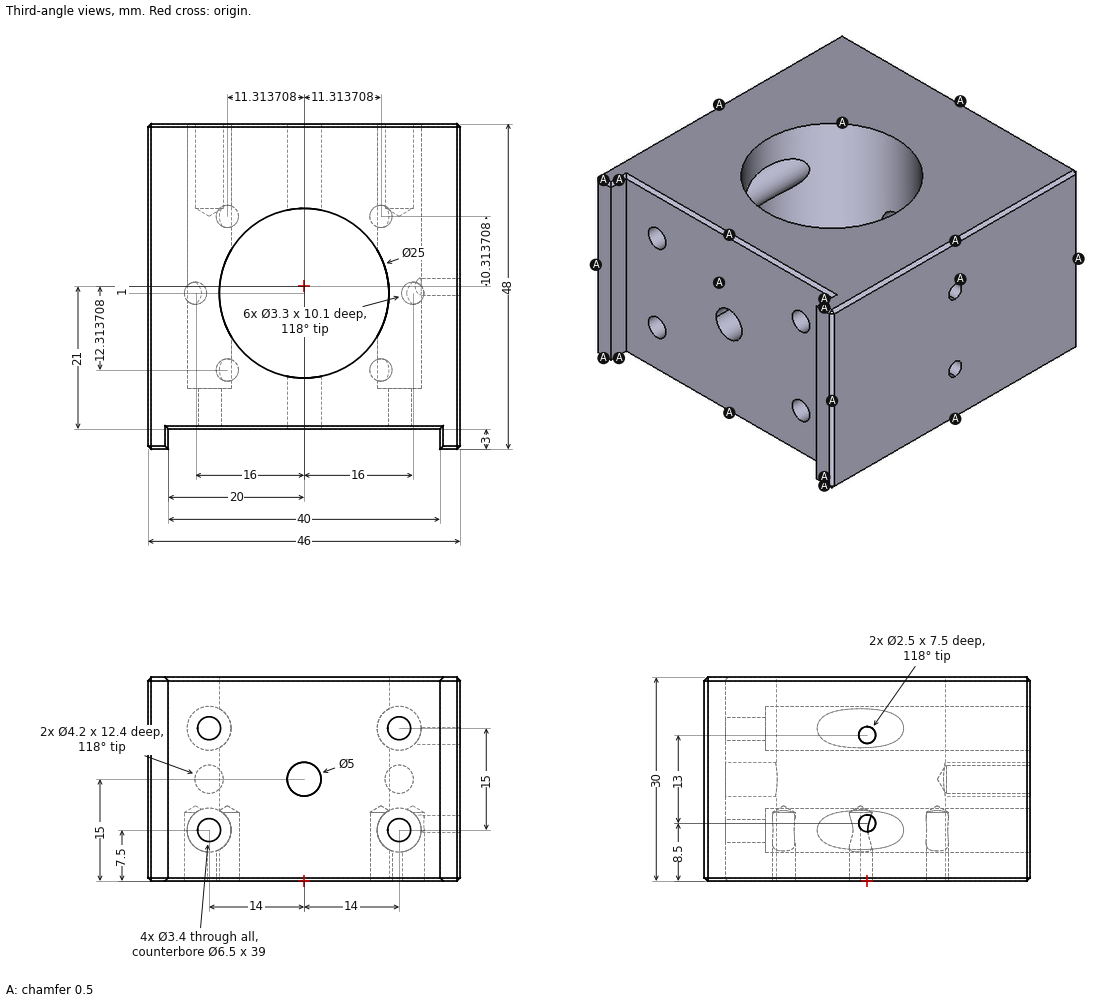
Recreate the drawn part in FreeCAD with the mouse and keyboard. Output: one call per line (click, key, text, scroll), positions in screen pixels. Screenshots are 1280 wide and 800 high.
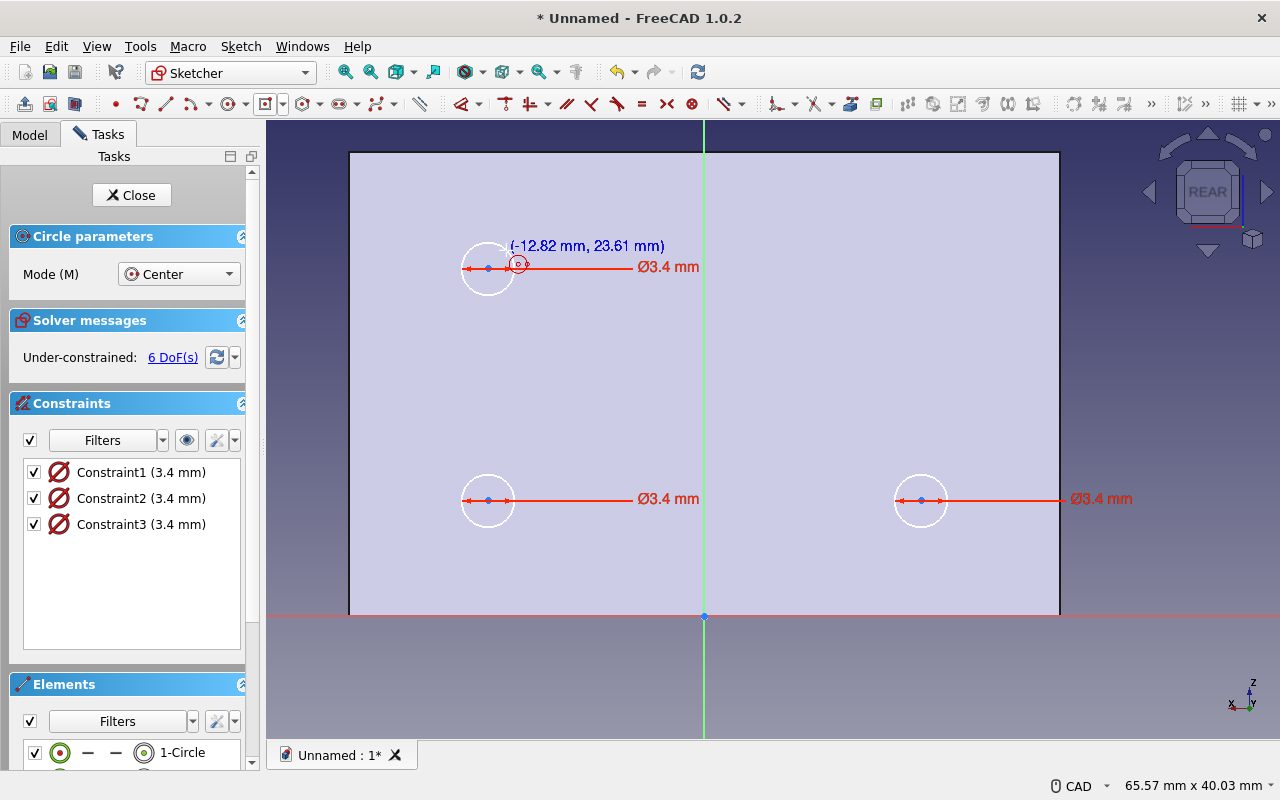
click(921, 268)
move(939, 250)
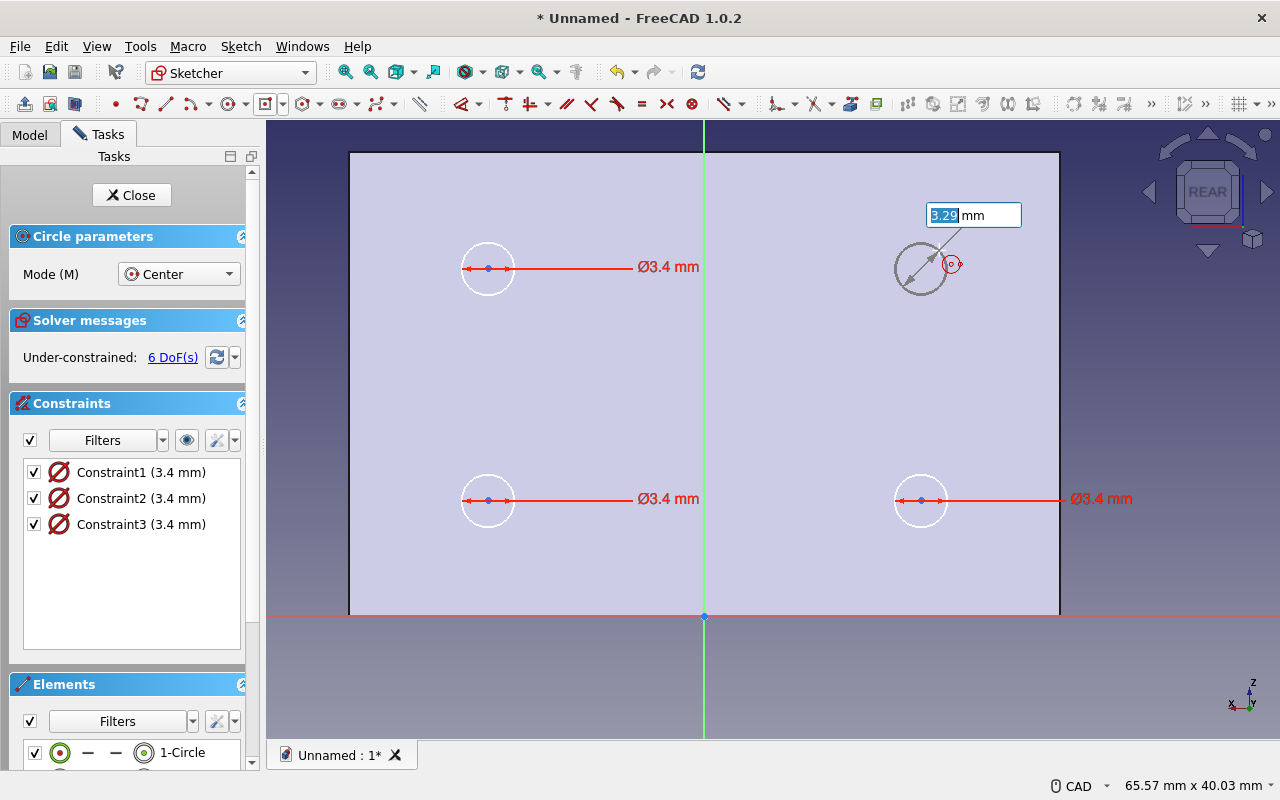
text(3.4)
key(Return)
key(Escape)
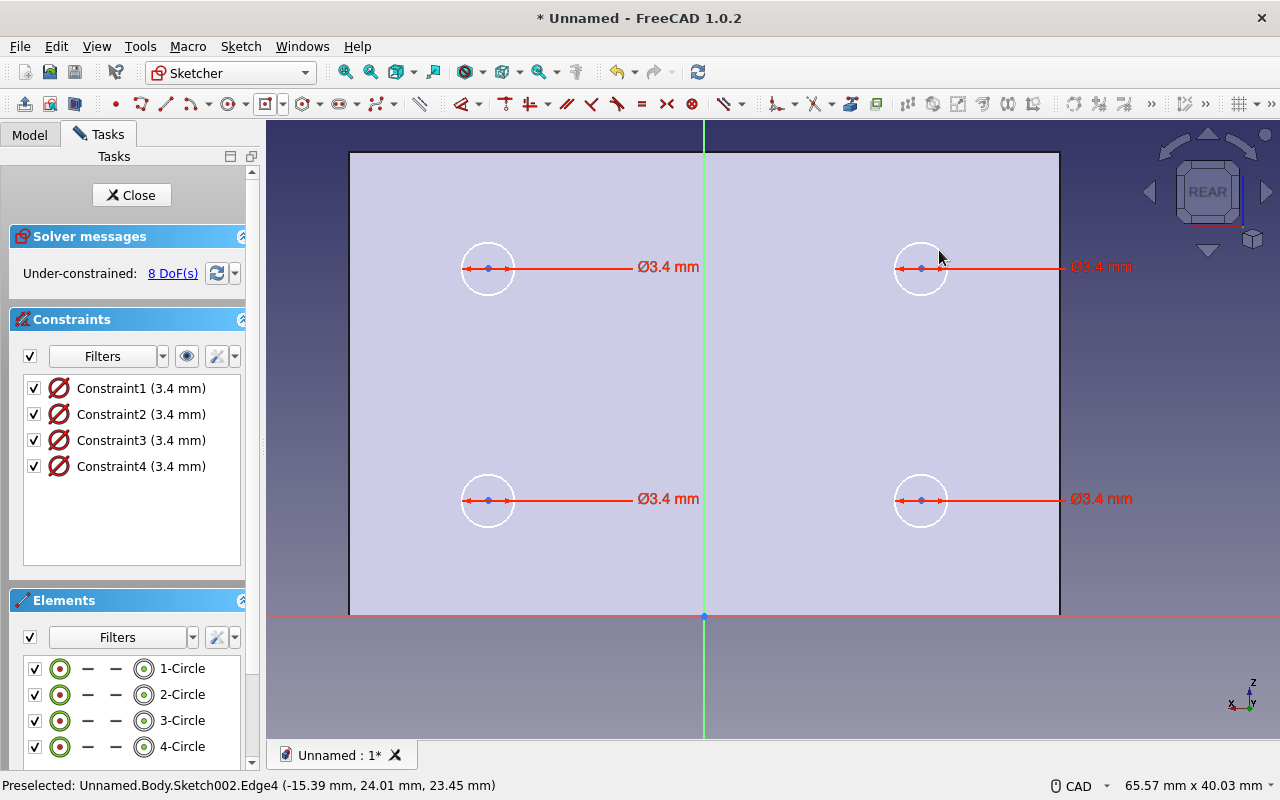
click(921, 501)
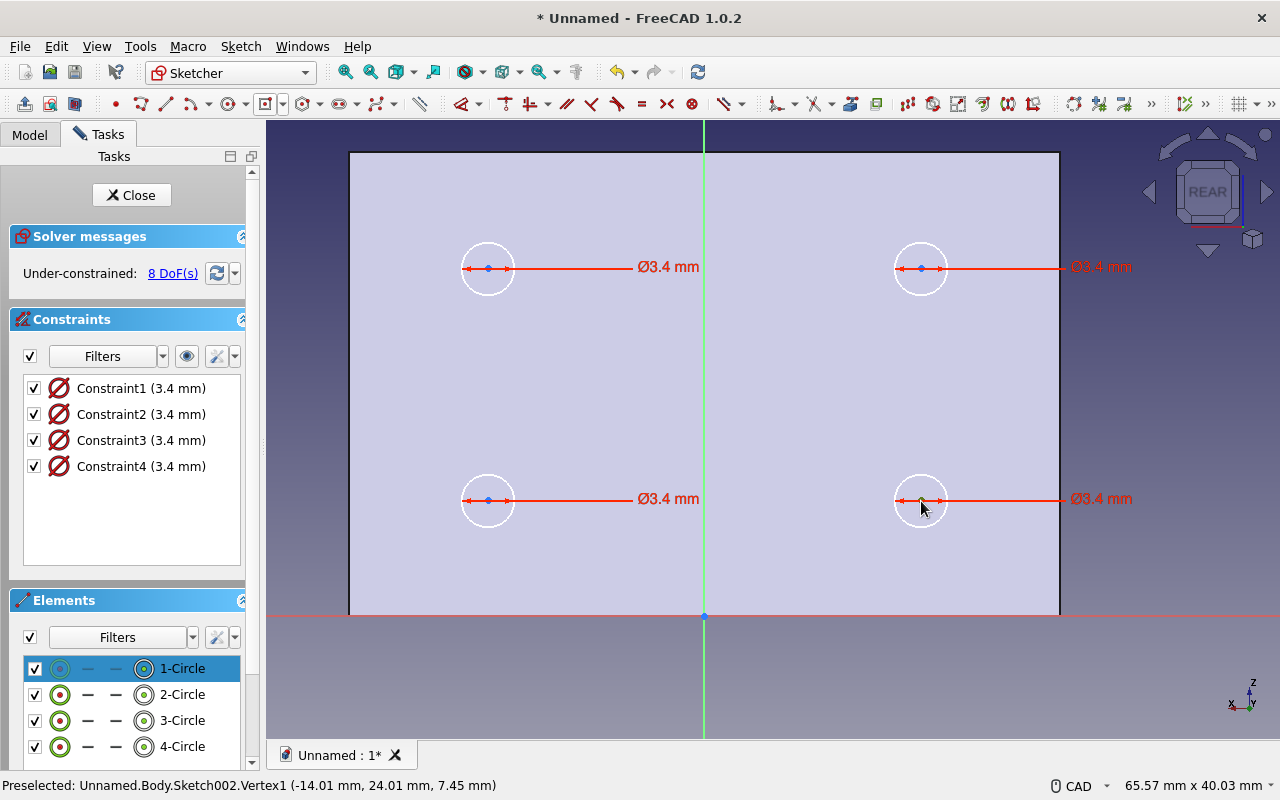
click(488, 501)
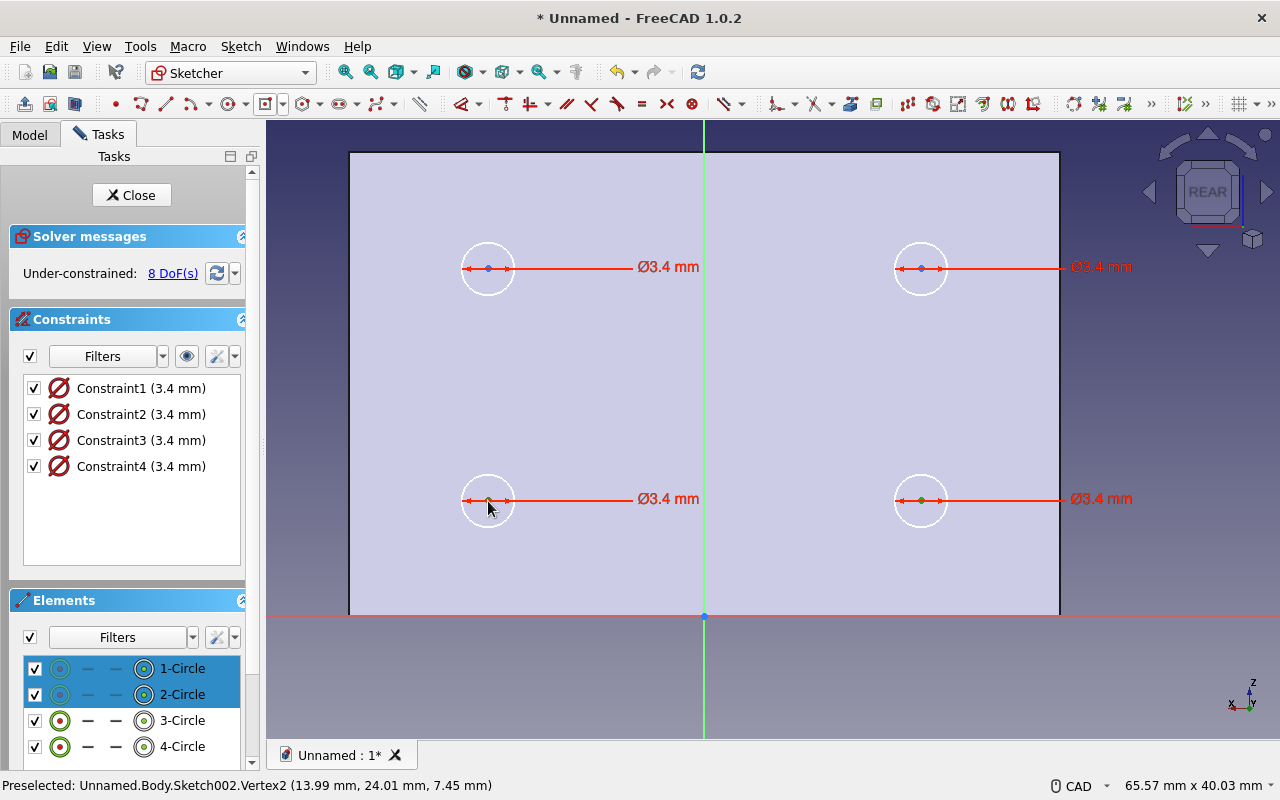
key(h)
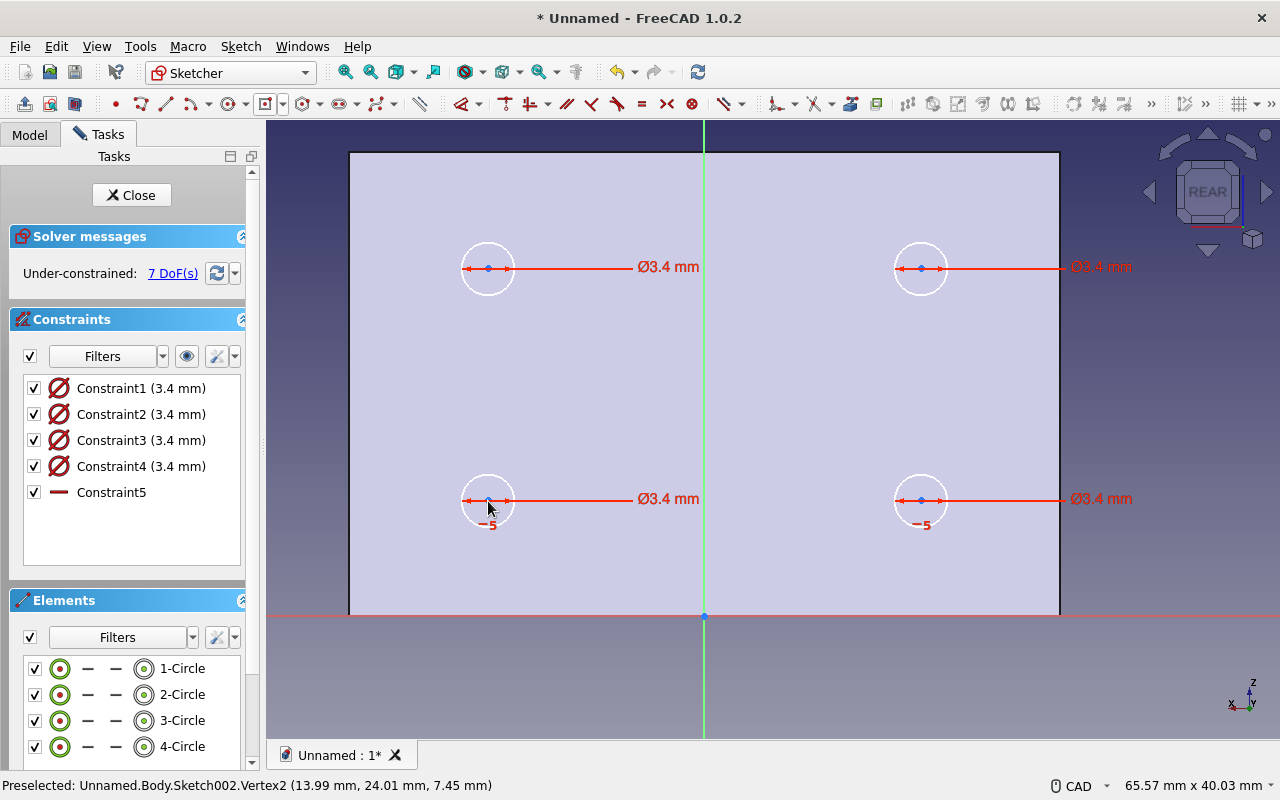
click(488, 501)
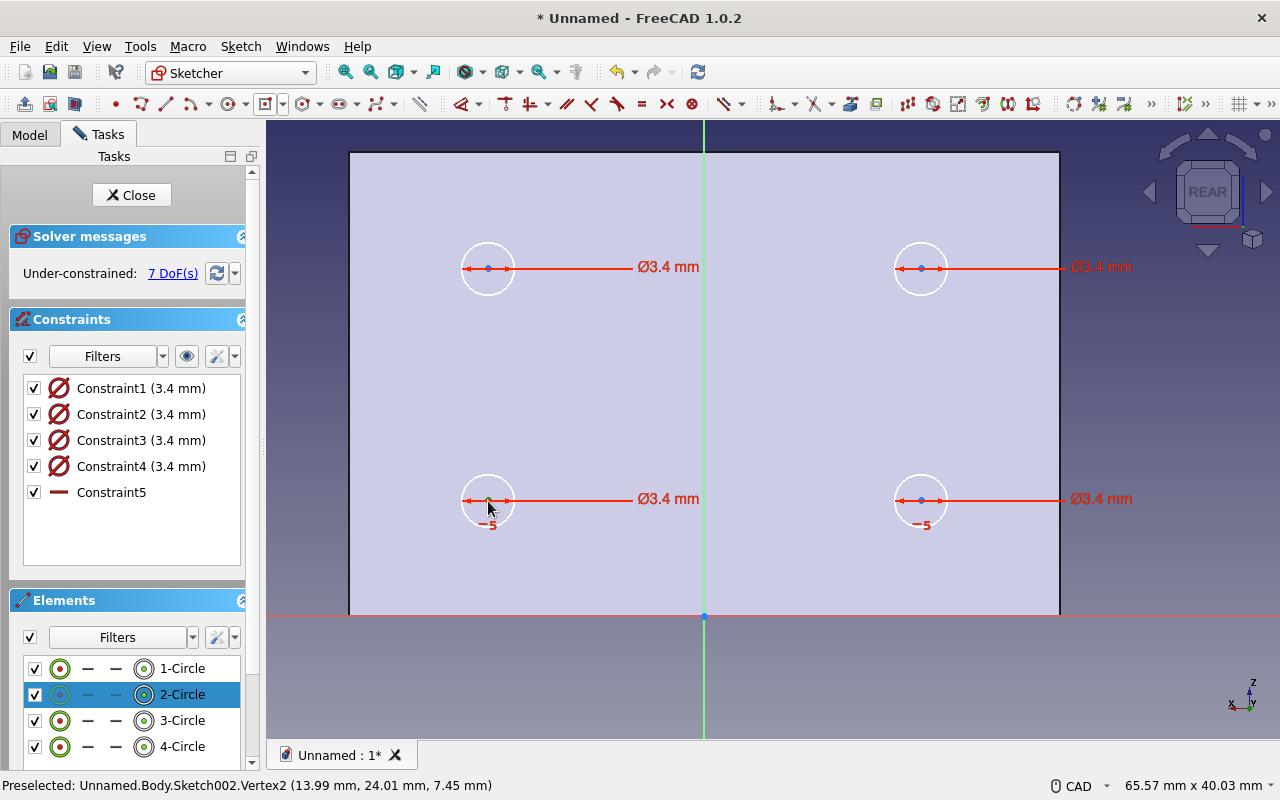
click(488, 269)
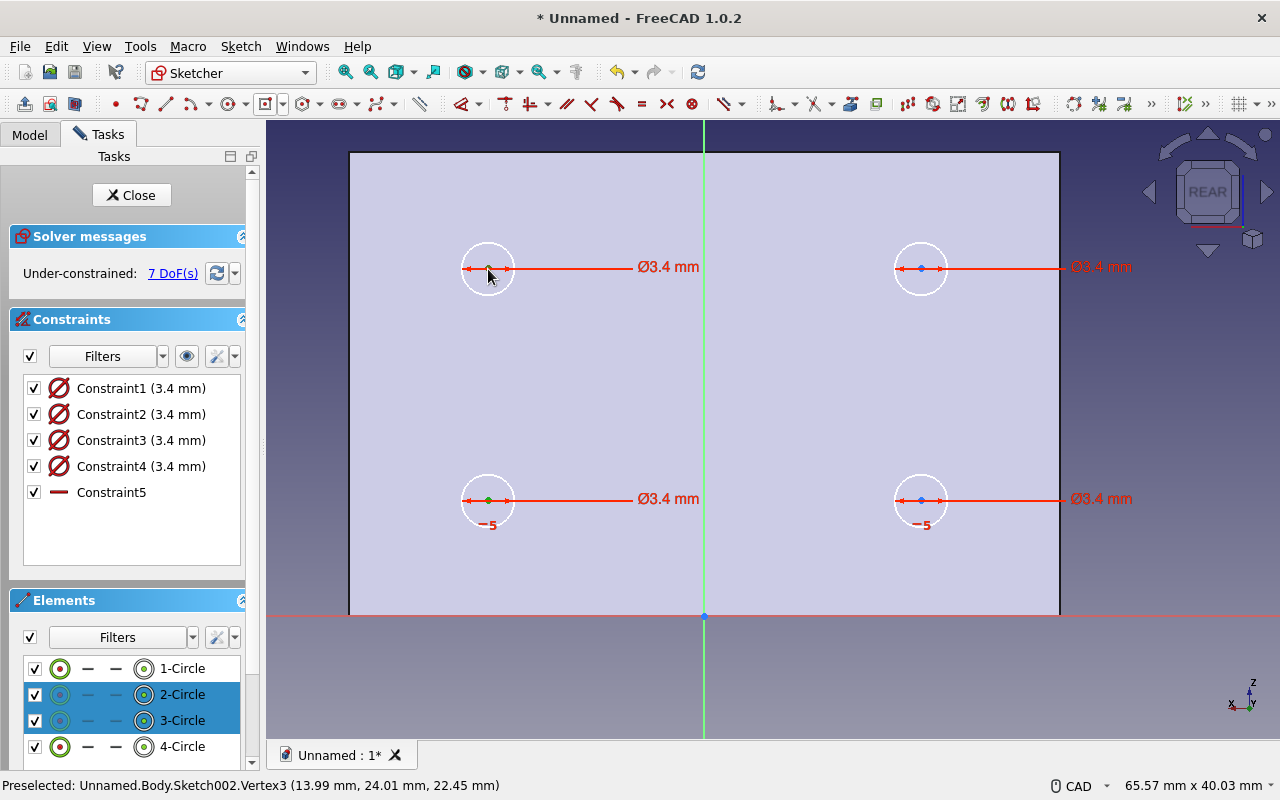
click(548, 104)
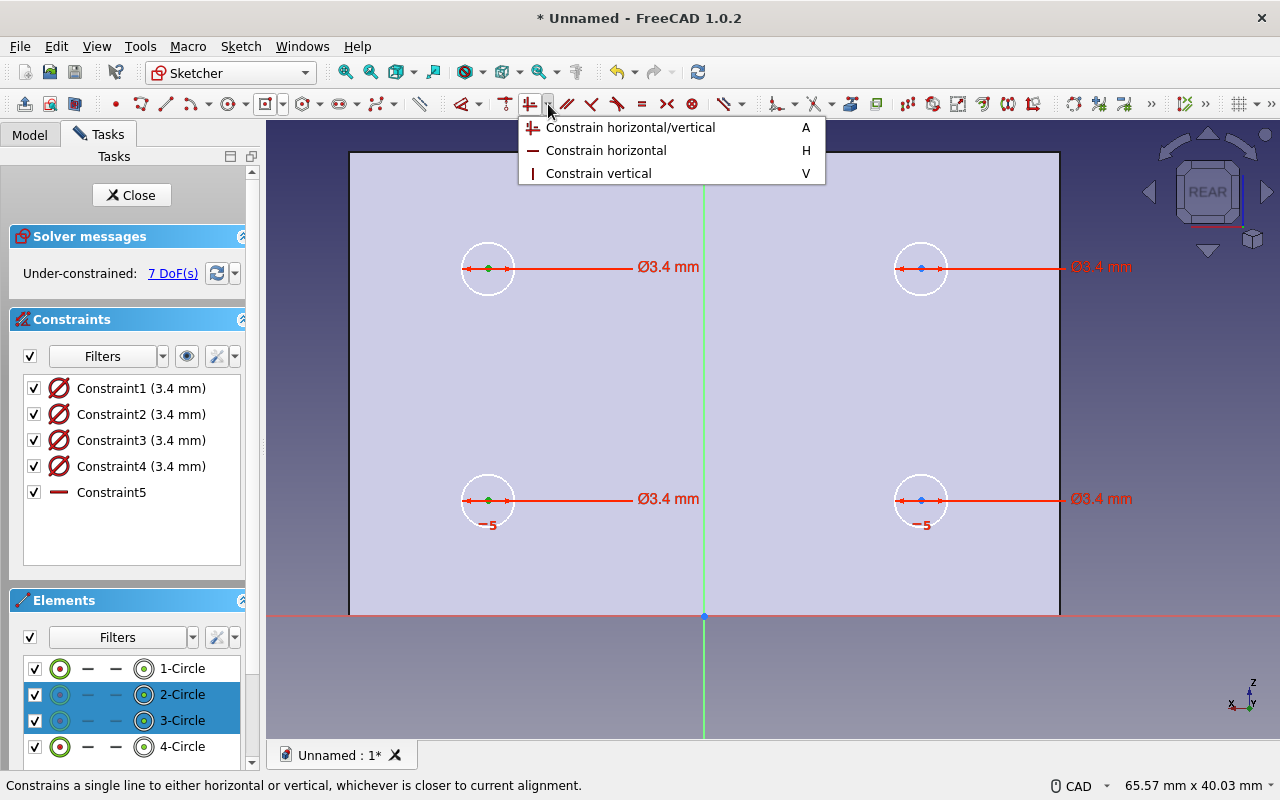
click(672, 174)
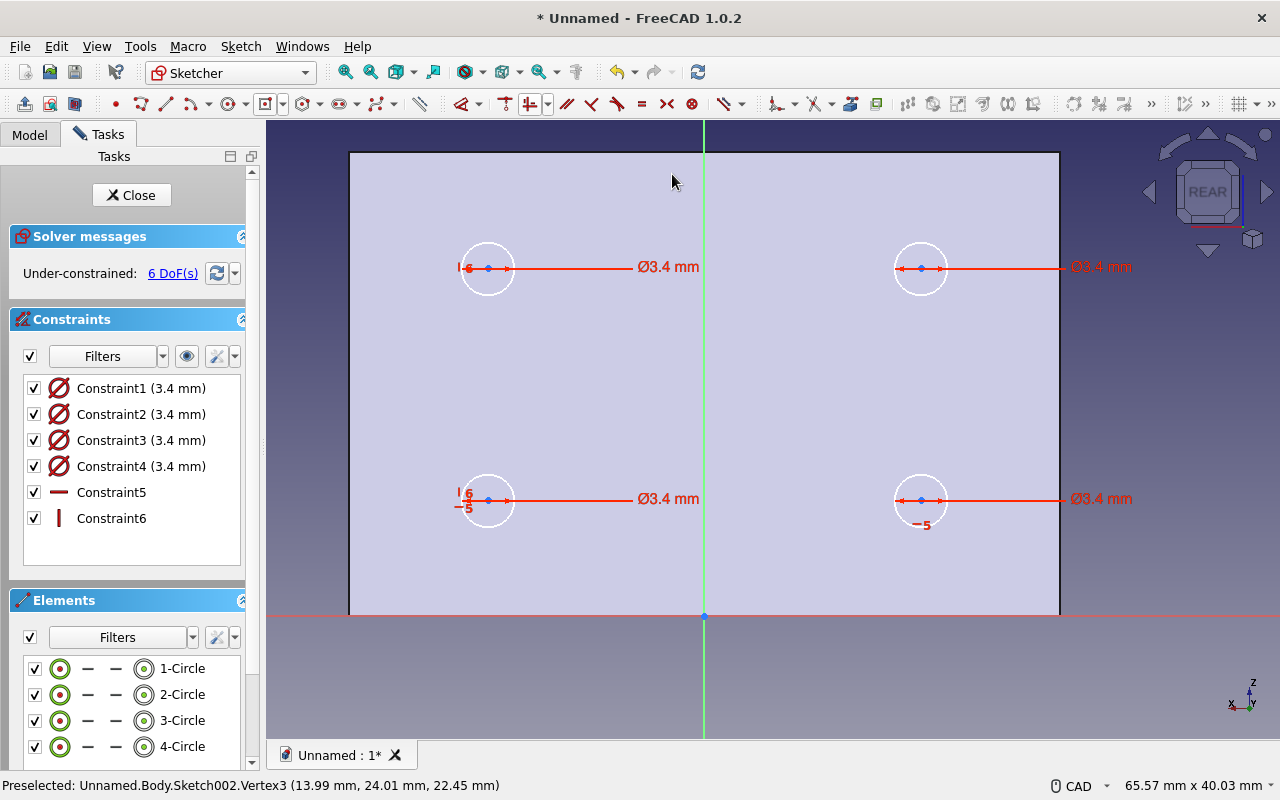
click(921, 501)